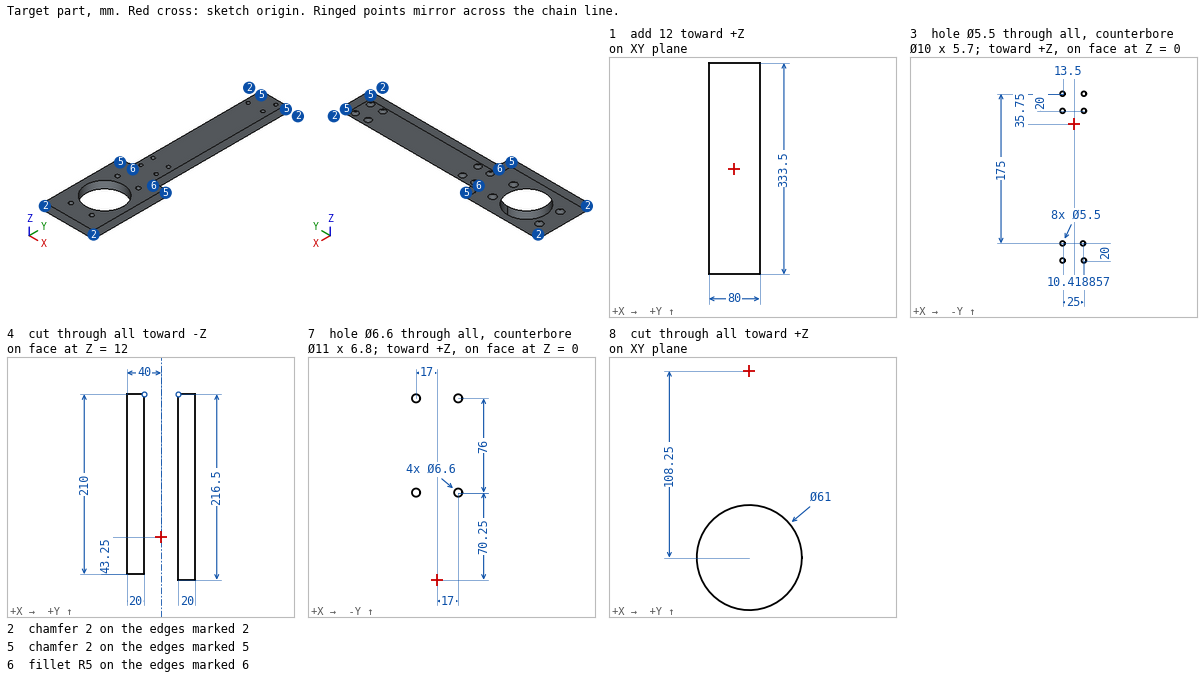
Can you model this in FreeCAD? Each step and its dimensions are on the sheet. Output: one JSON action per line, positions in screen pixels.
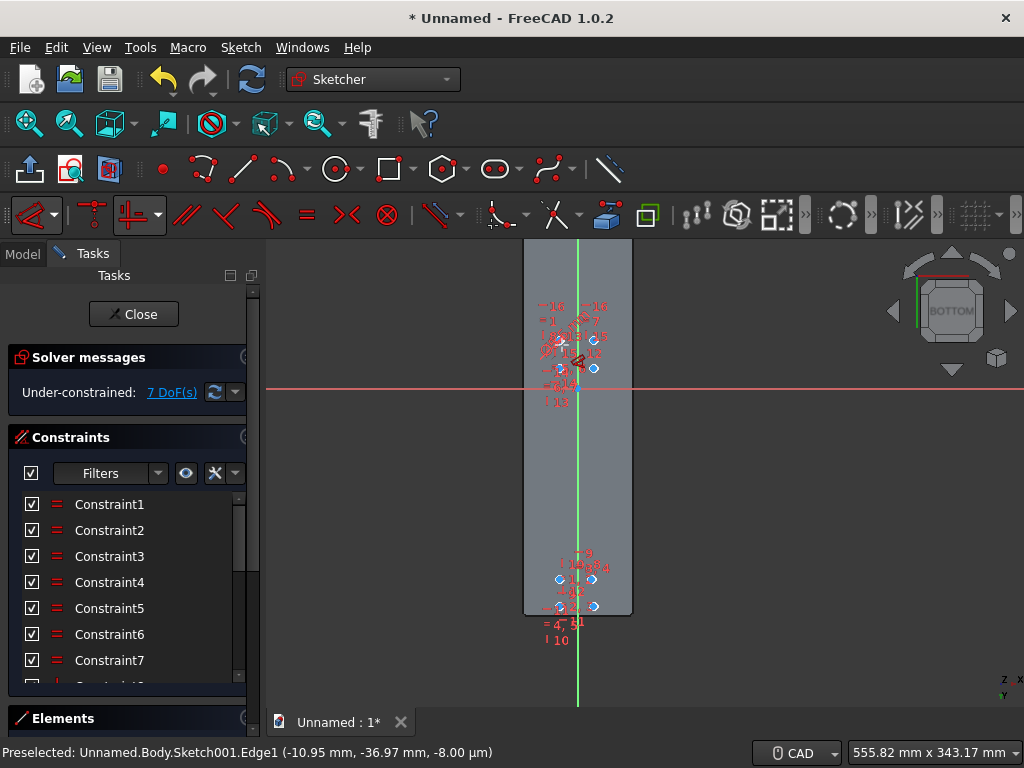
{"action": "left_click", "coordinate": [560, 580]}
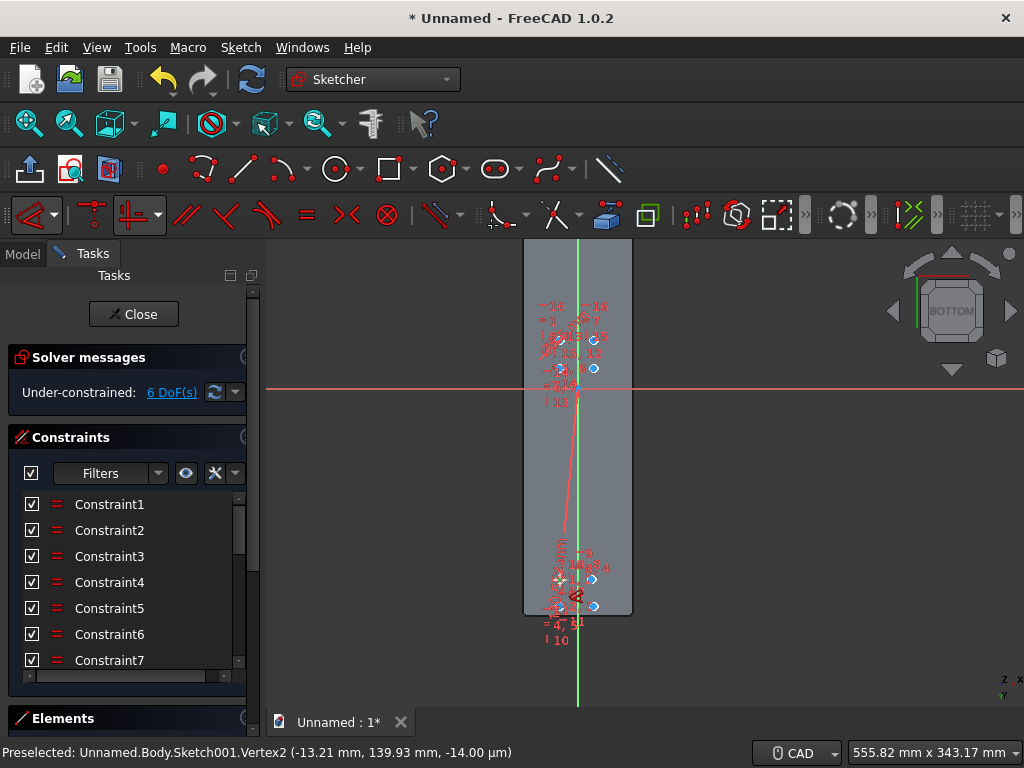
{"action": "left_click", "coordinate": [594, 607]}
{"action": "left_click", "coordinate": [569, 641]}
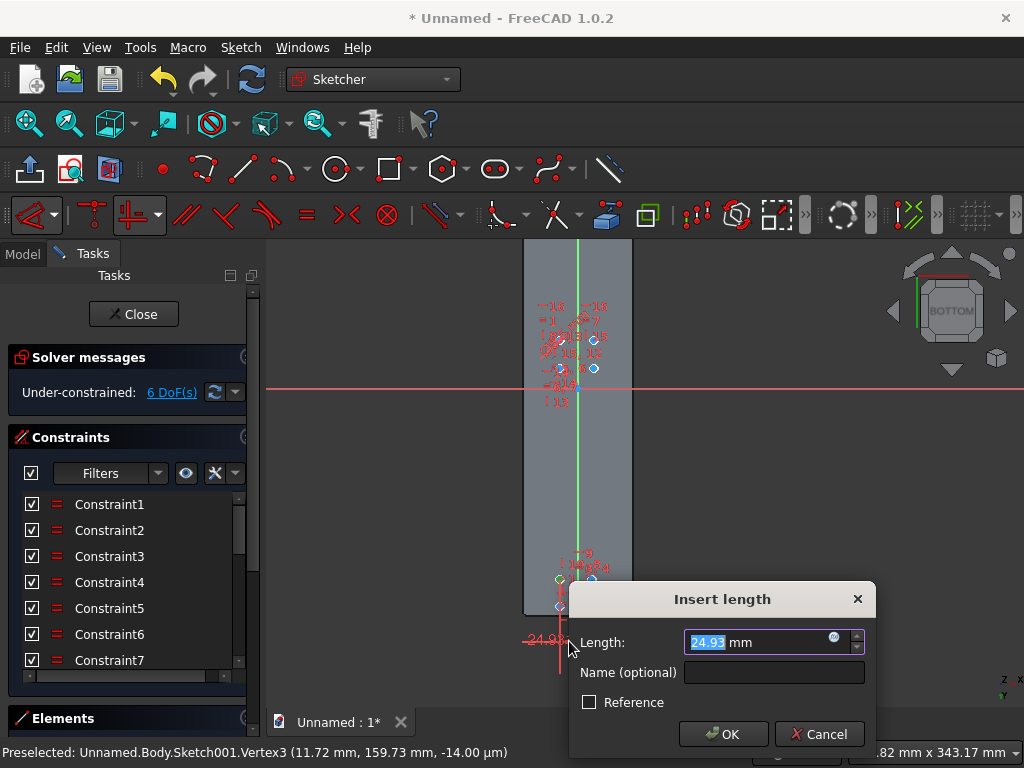
{"action": "type", "text": "25"}
{"action": "key", "text": "Return"}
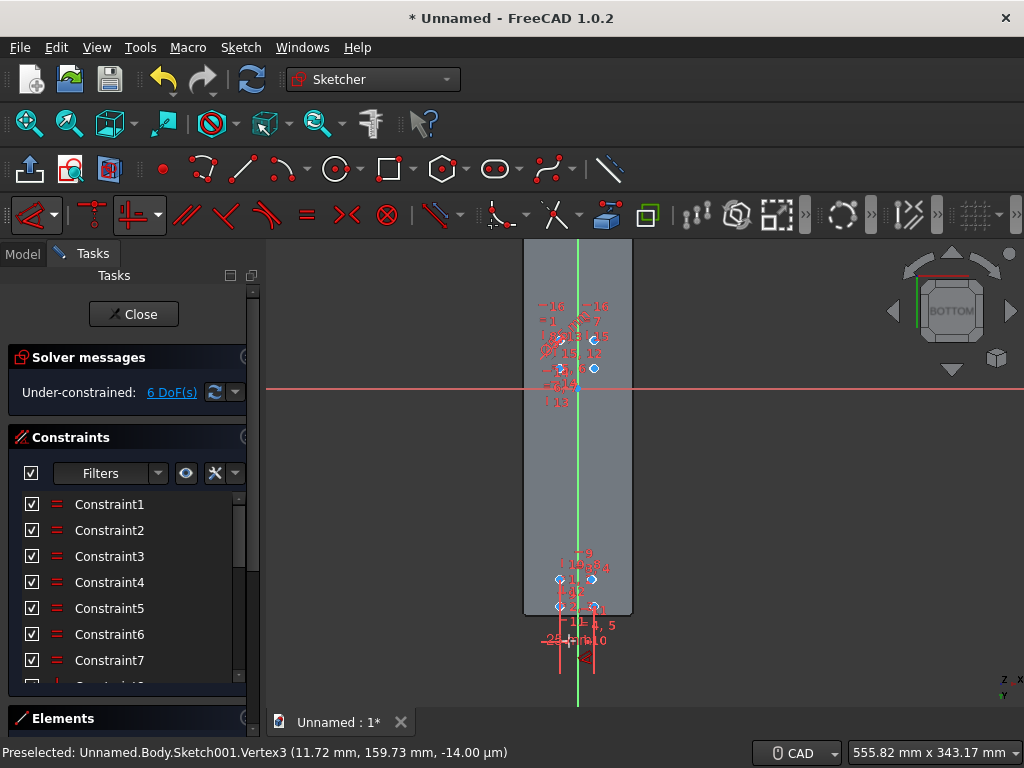
{"action": "scroll", "coordinate": [560, 580], "scroll_direction": "up", "scroll_amount": 2}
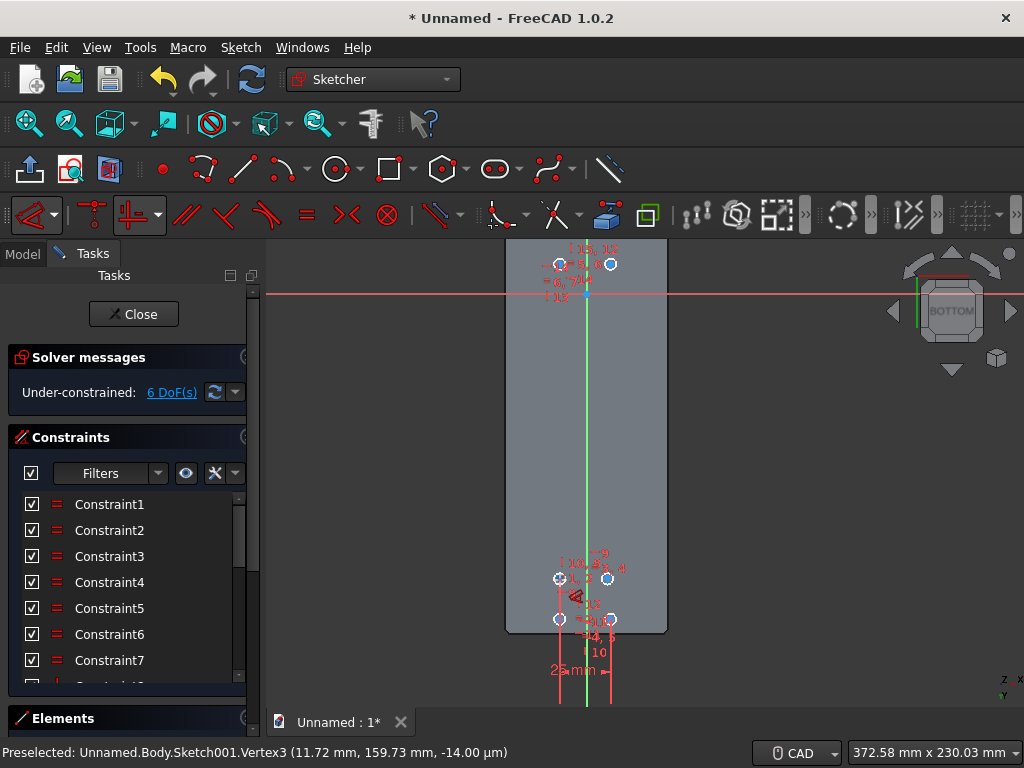
{"action": "left_click", "coordinate": [560, 579]}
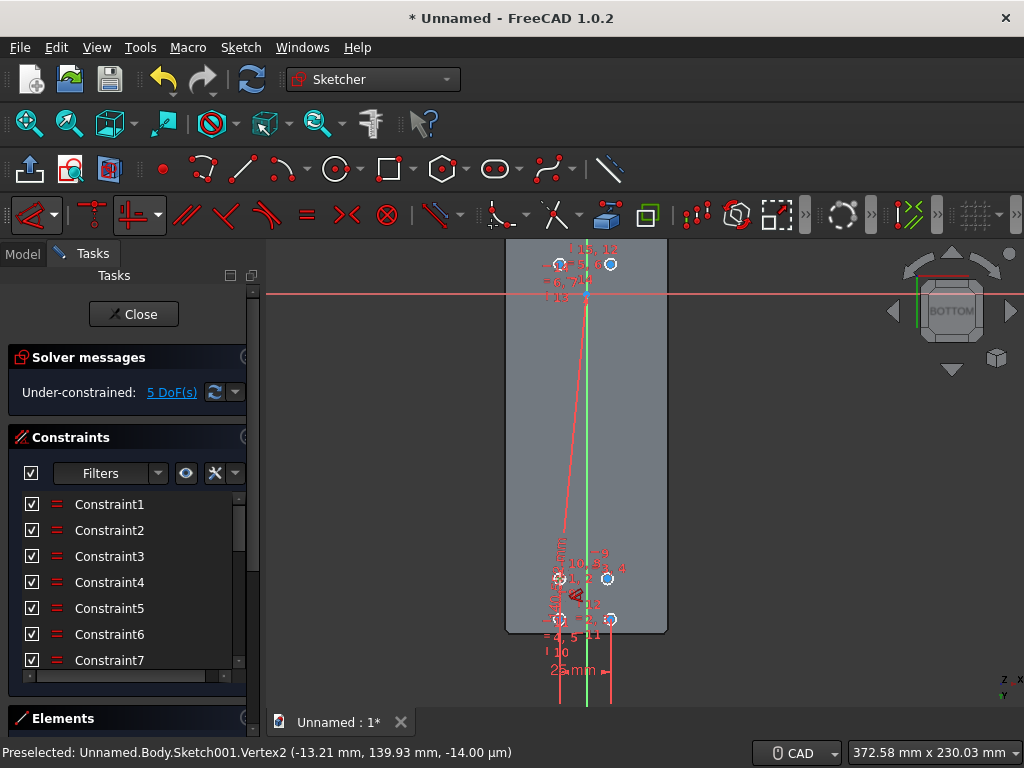
{"action": "left_click", "coordinate": [611, 619]}
{"action": "left_click", "coordinate": [645, 599]}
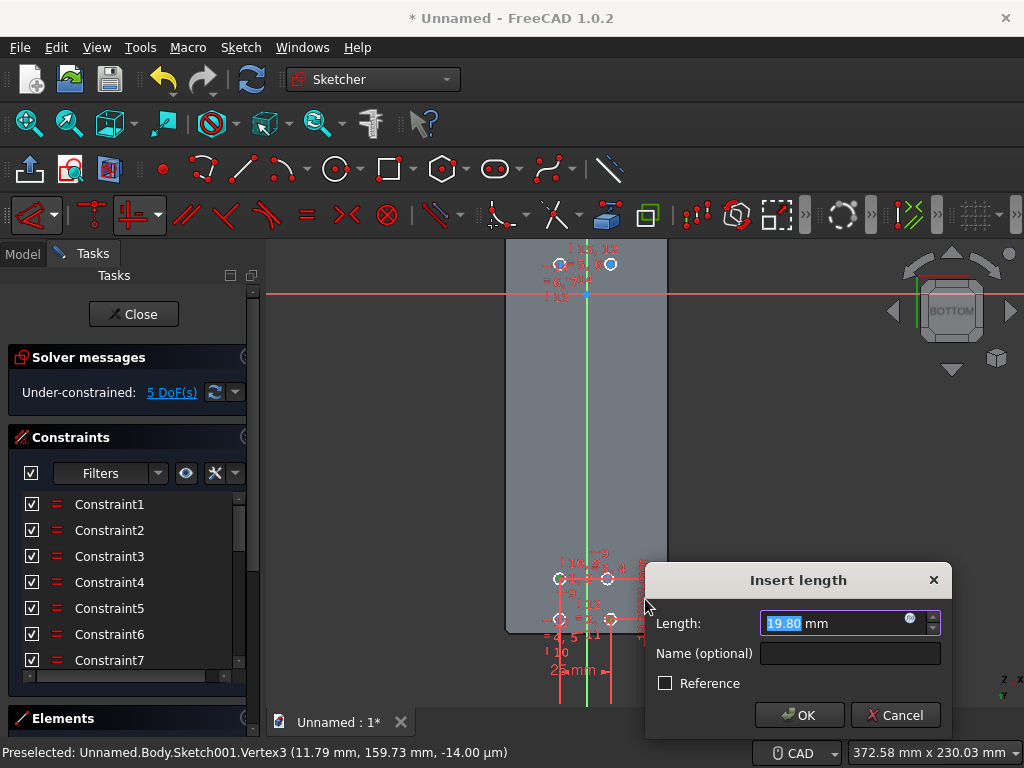
{"action": "type", "text": "20"}
{"action": "key", "text": "Return"}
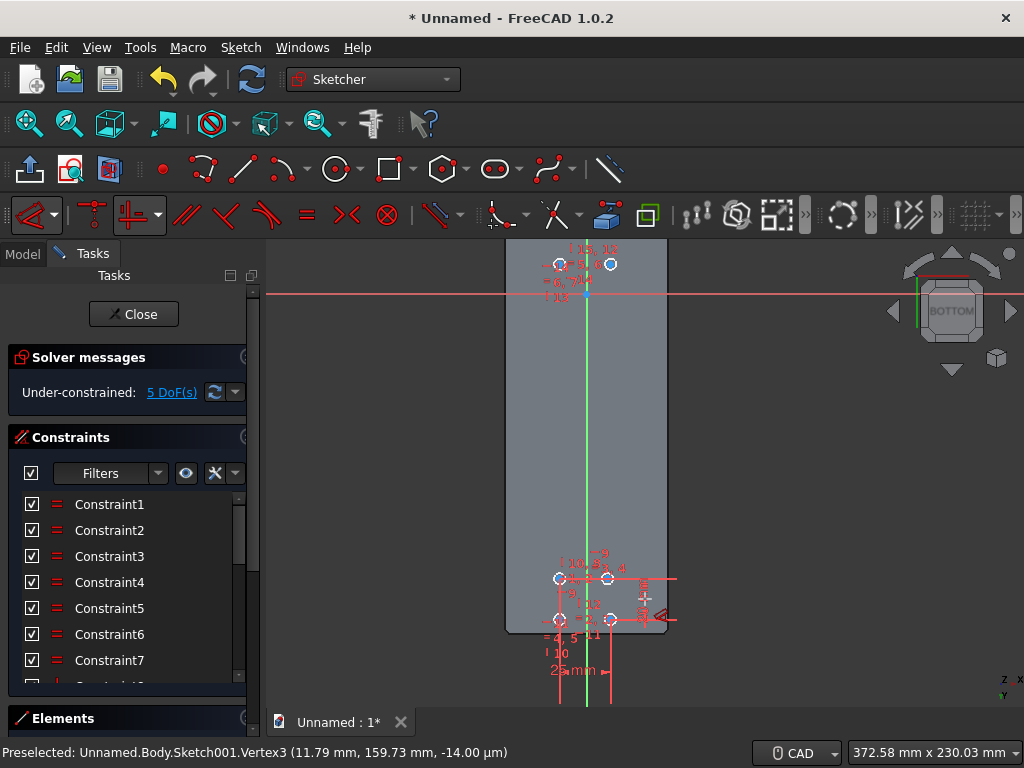
{"action": "scroll", "coordinate": [560, 581], "scroll_direction": "down", "scroll_amount": 2}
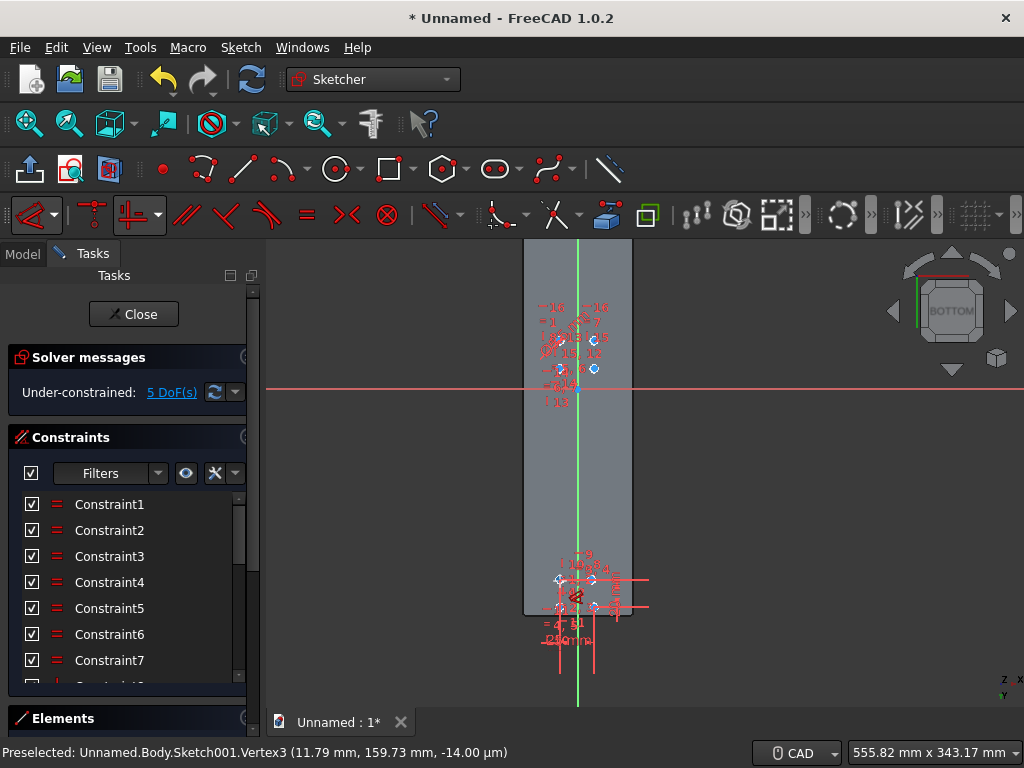
{"action": "scroll", "coordinate": [560, 341], "scroll_direction": "up", "scroll_amount": 2}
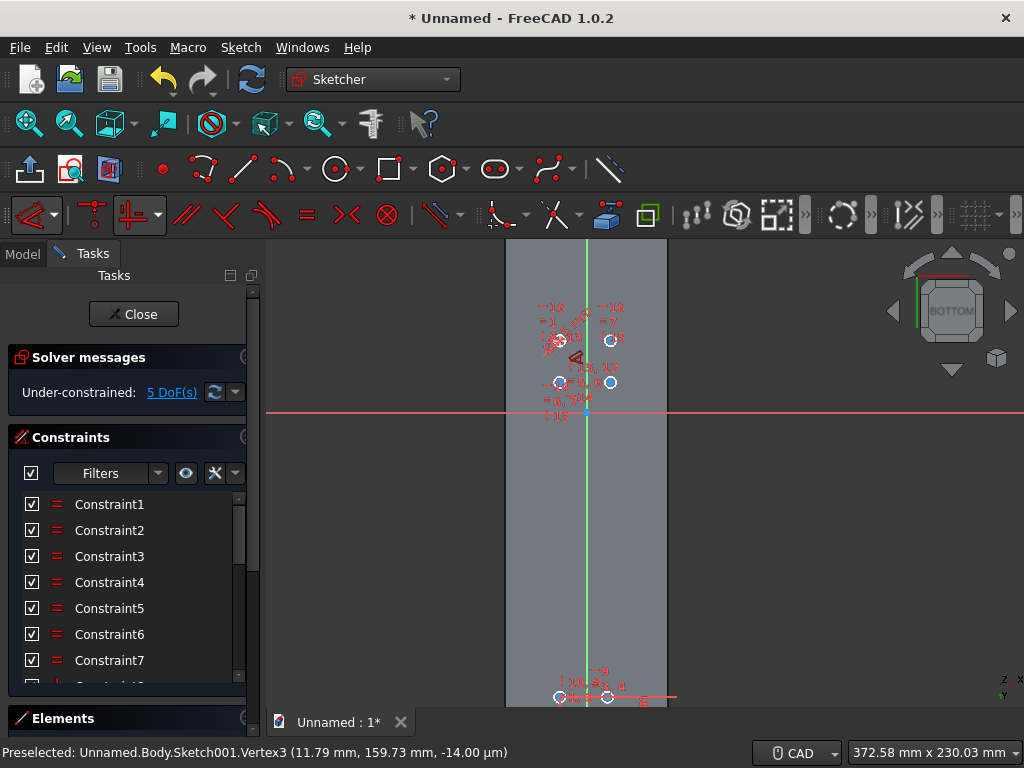
{"action": "left_click", "coordinate": [560, 341]}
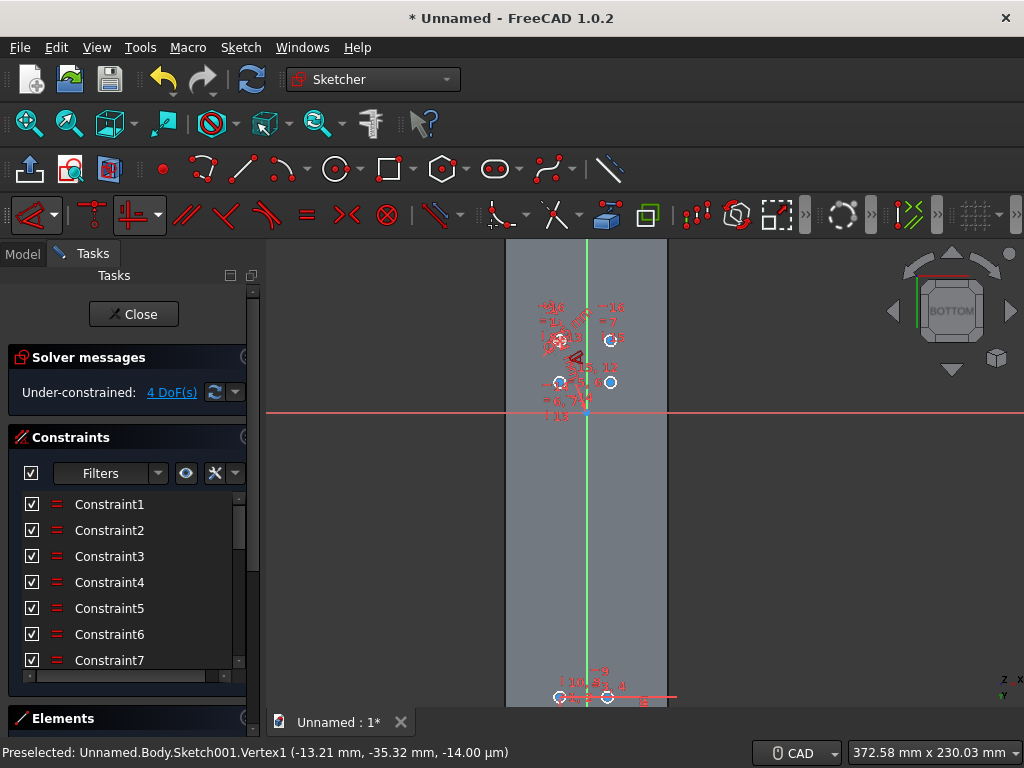
{"action": "left_click", "coordinate": [611, 383]}
{"action": "left_click", "coordinate": [645, 362]}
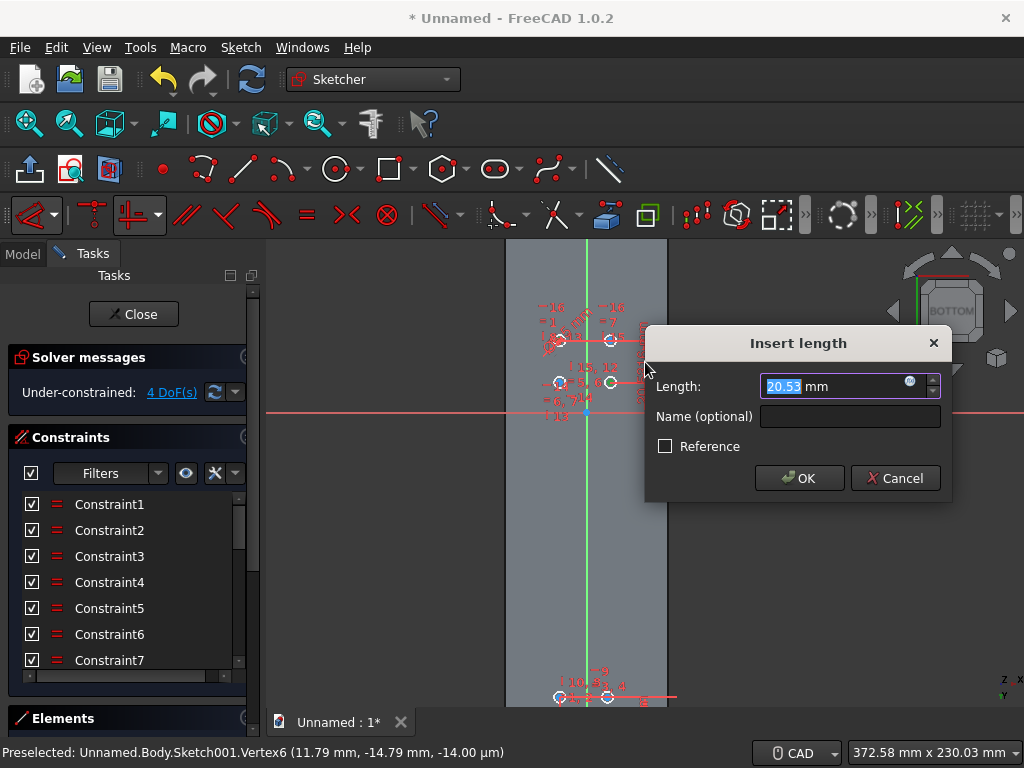
{"action": "type", "text": "20"}
{"action": "key", "text": "Return"}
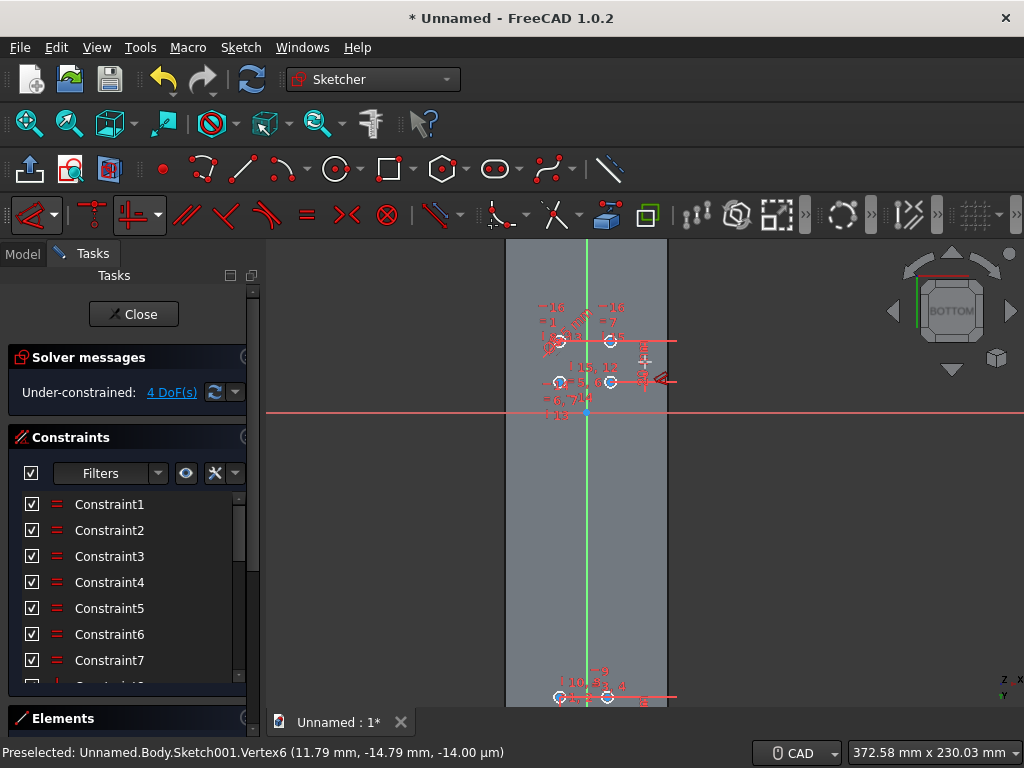
{"action": "scroll", "coordinate": [560, 341], "scroll_direction": "up", "scroll_amount": 2}